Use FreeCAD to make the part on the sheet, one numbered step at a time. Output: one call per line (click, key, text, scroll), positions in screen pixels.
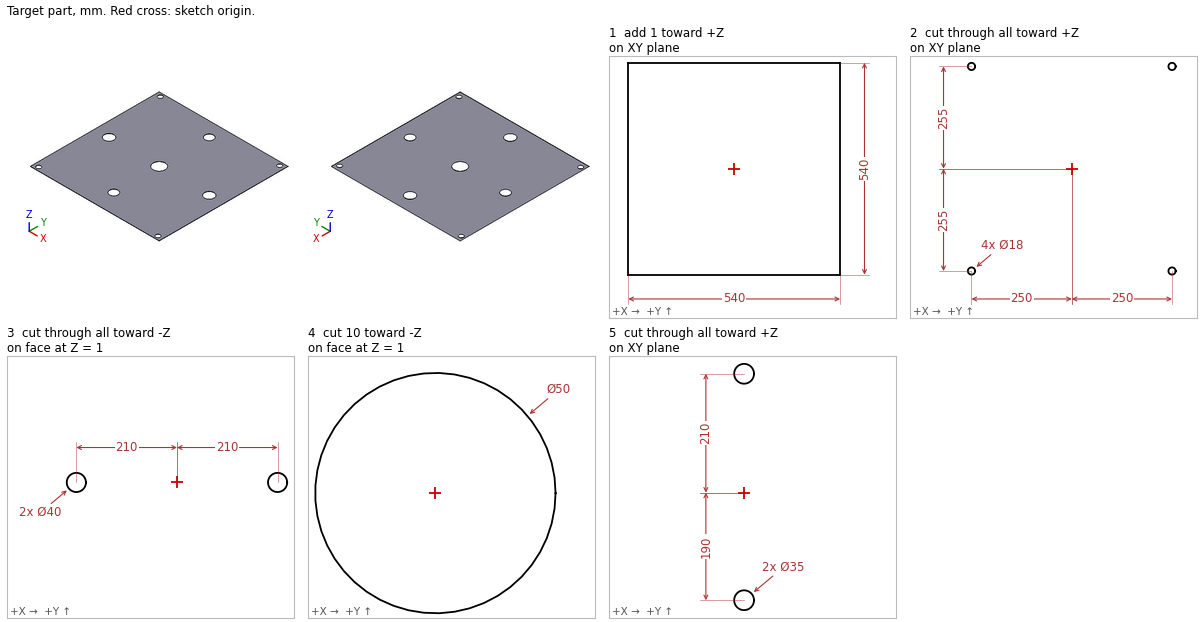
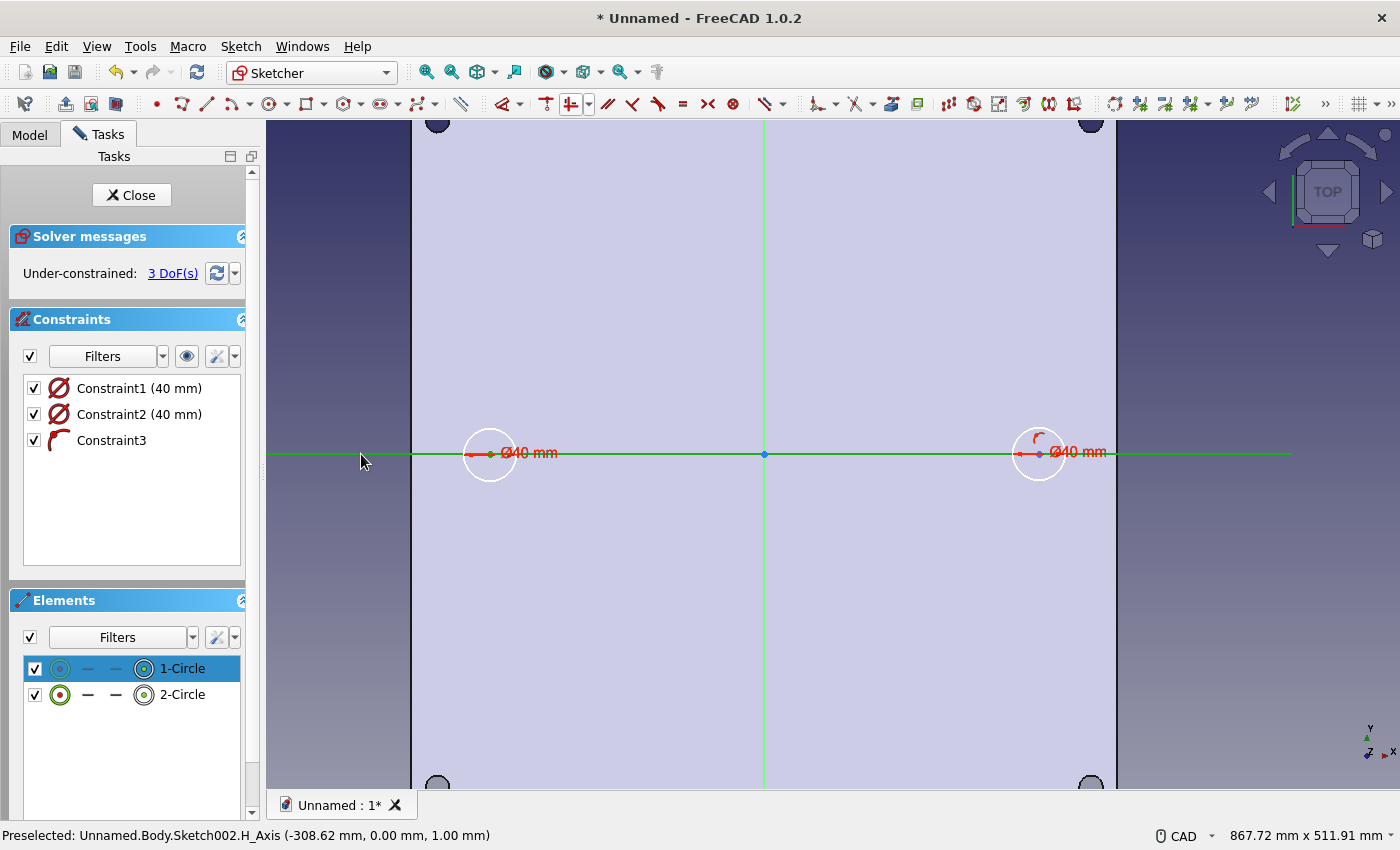
key(c)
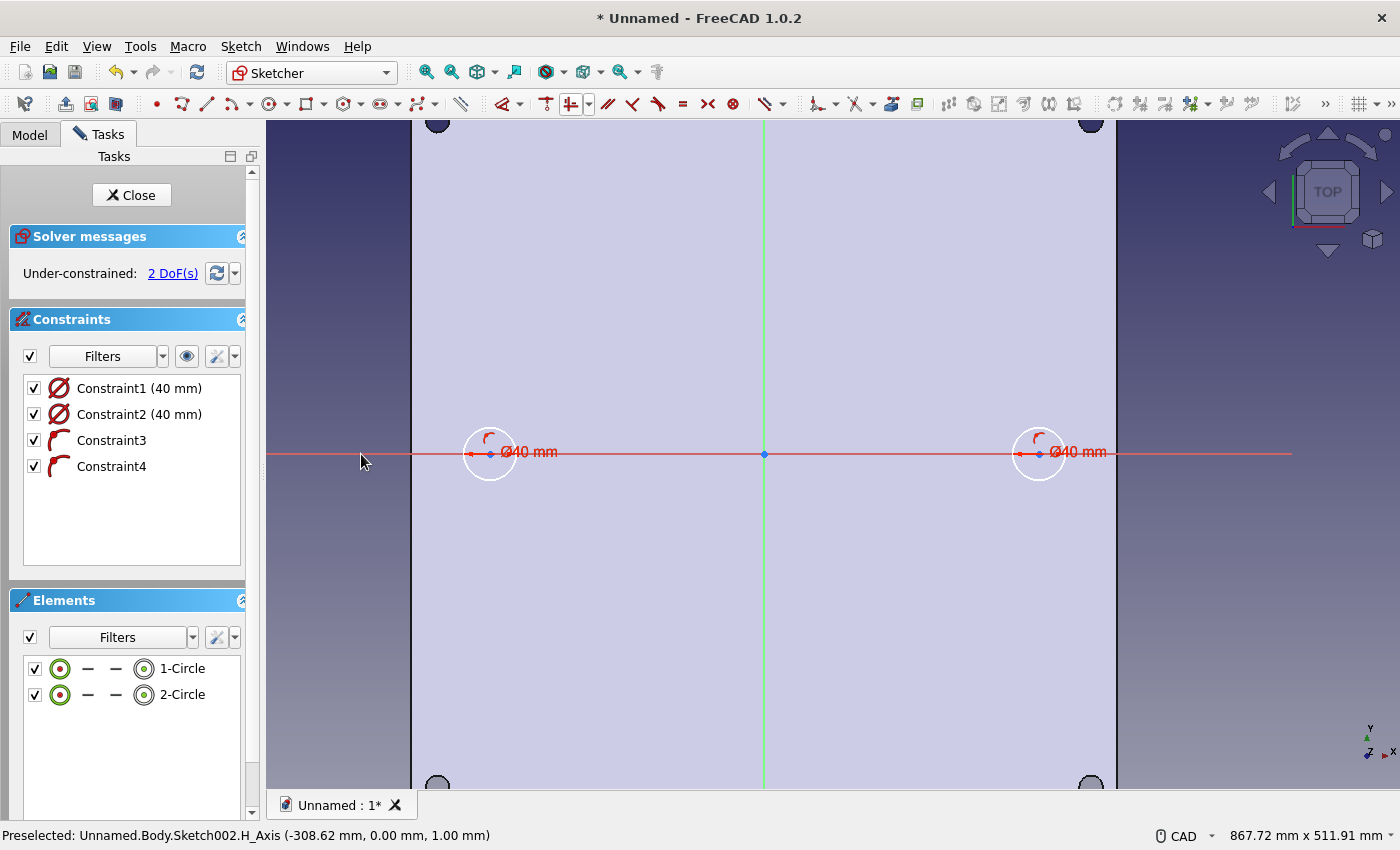
key(d)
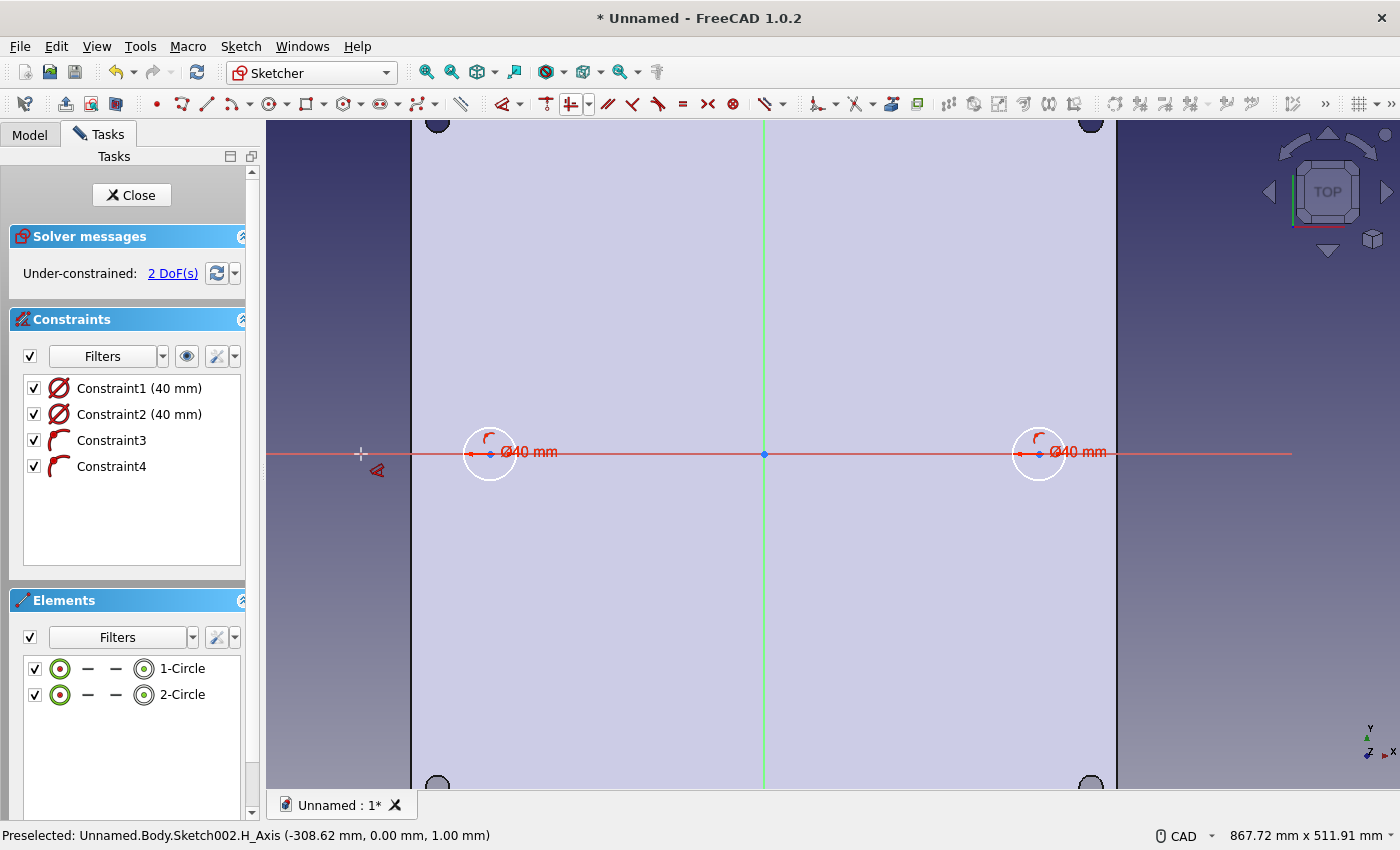
click(490, 454)
click(627, 488)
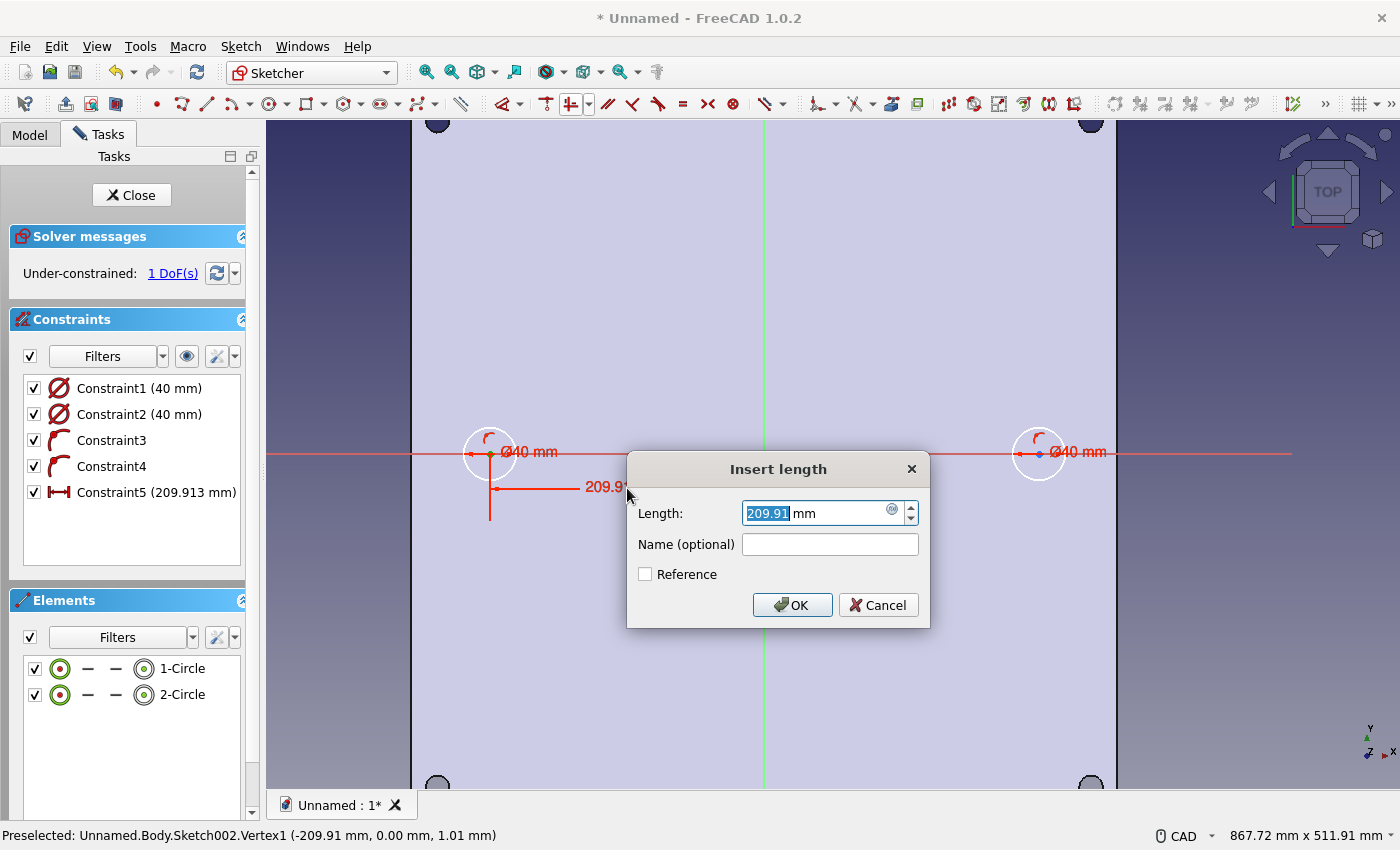
text(210)
key(Return)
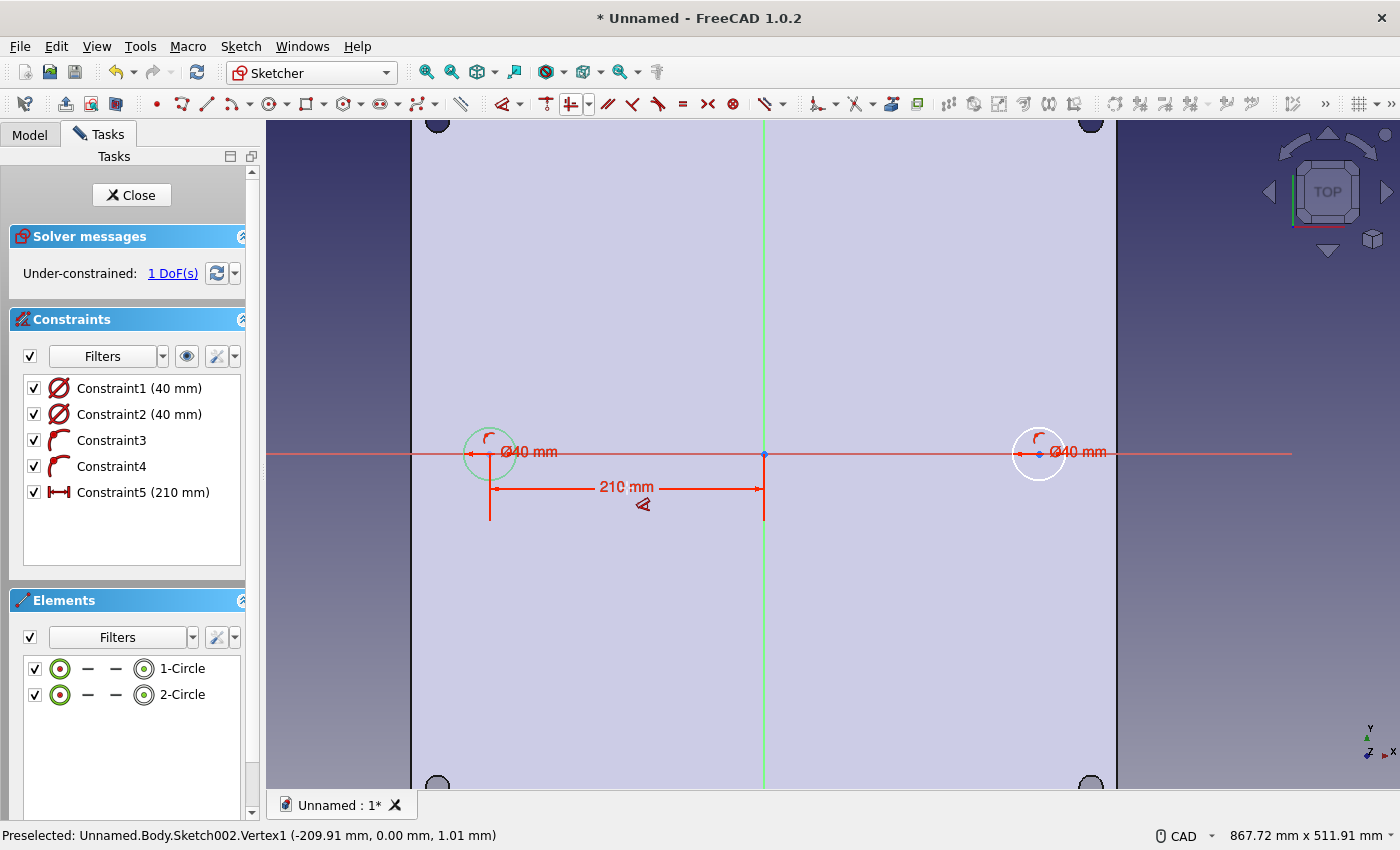
click(1039, 454)
click(902, 488)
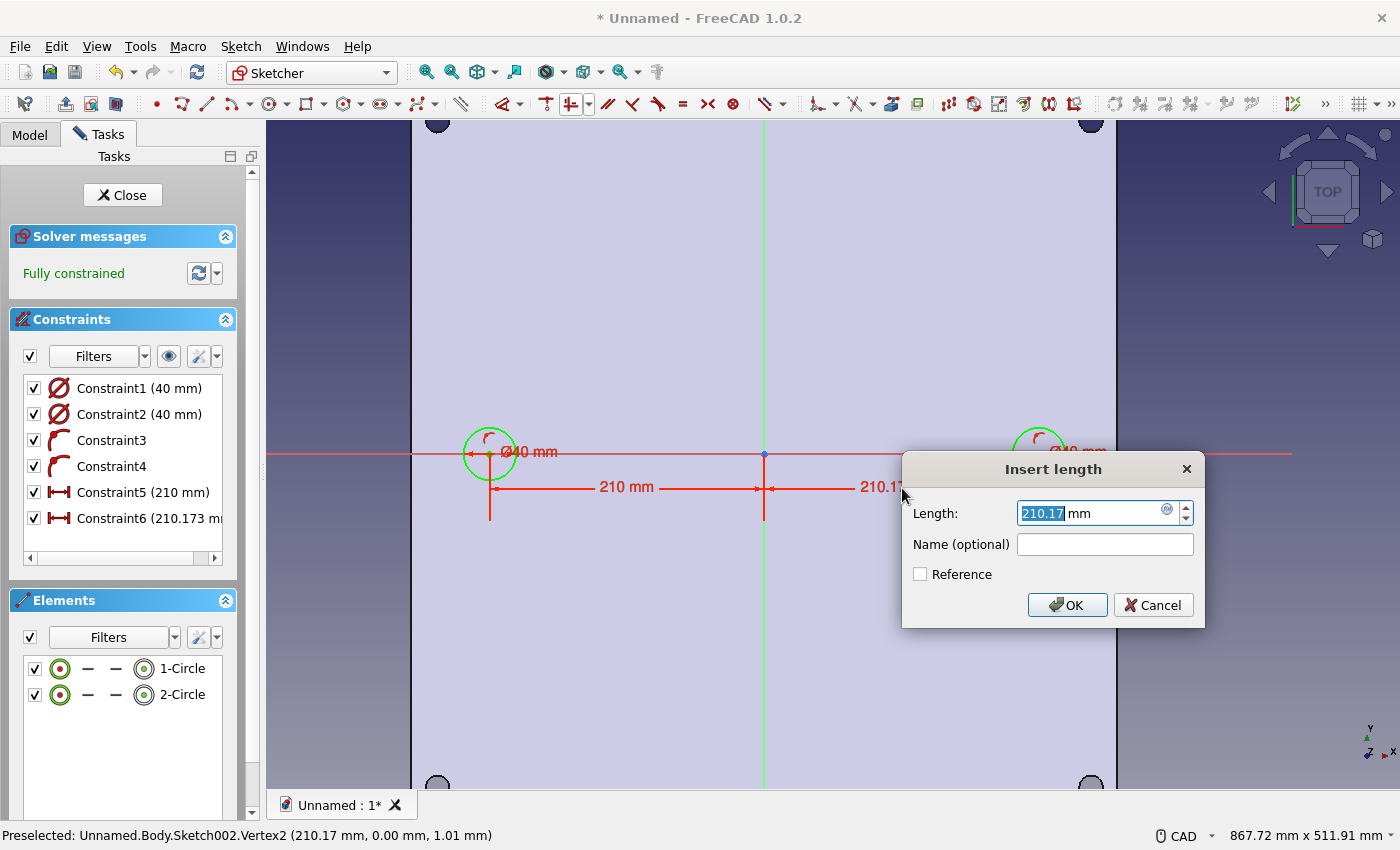
text(210)
key(Return)
key(Escape)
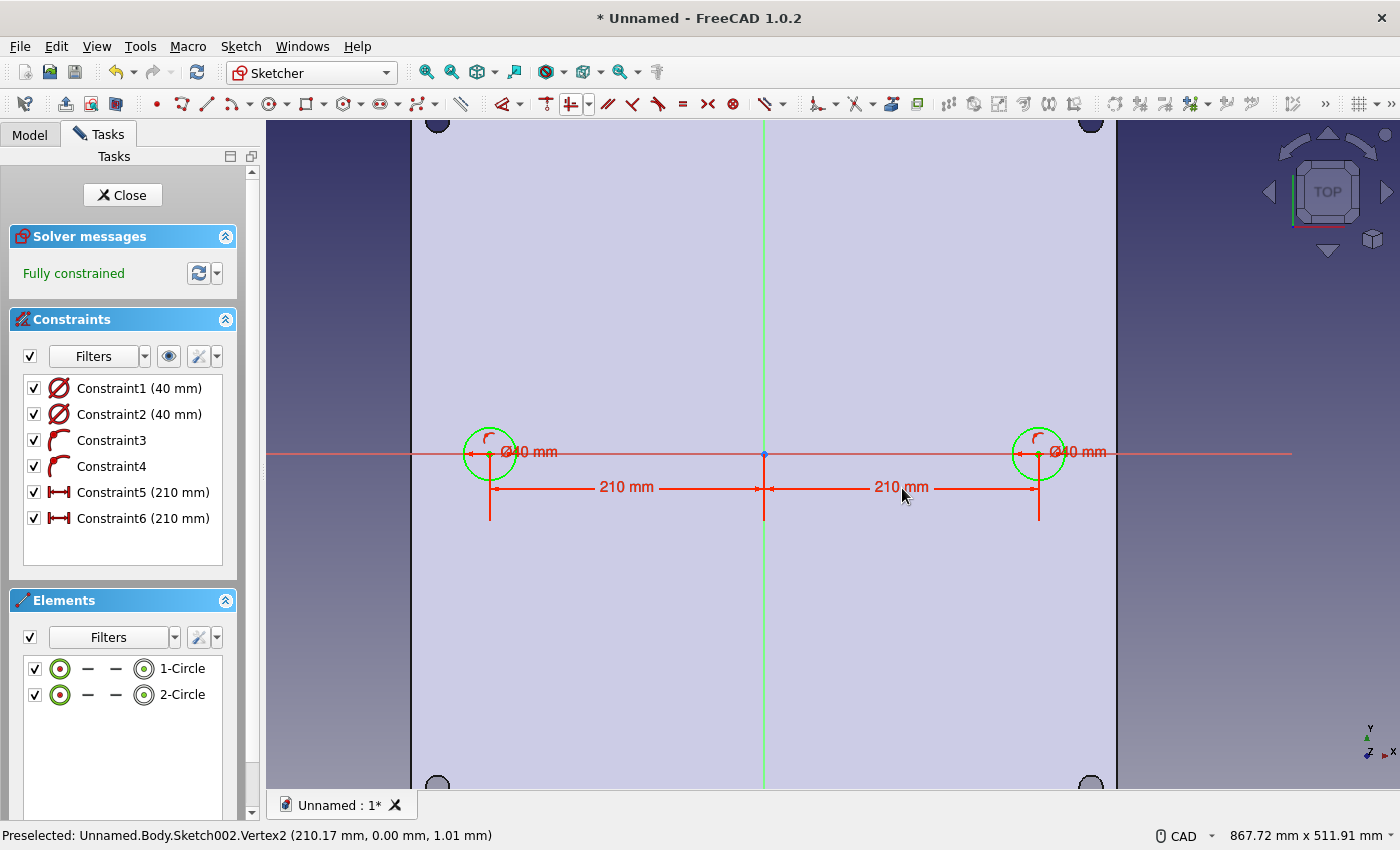
click(123, 195)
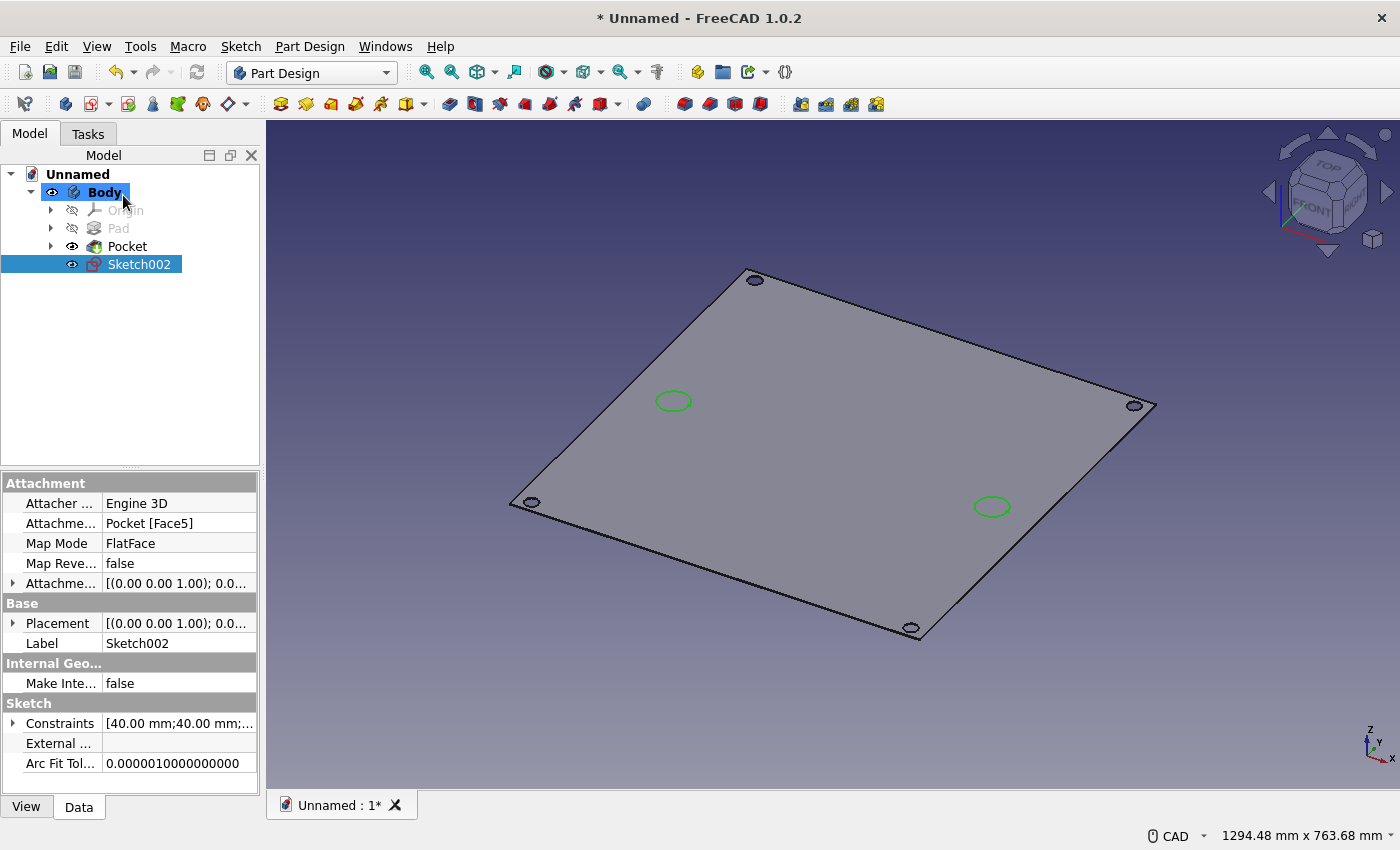
click(450, 104)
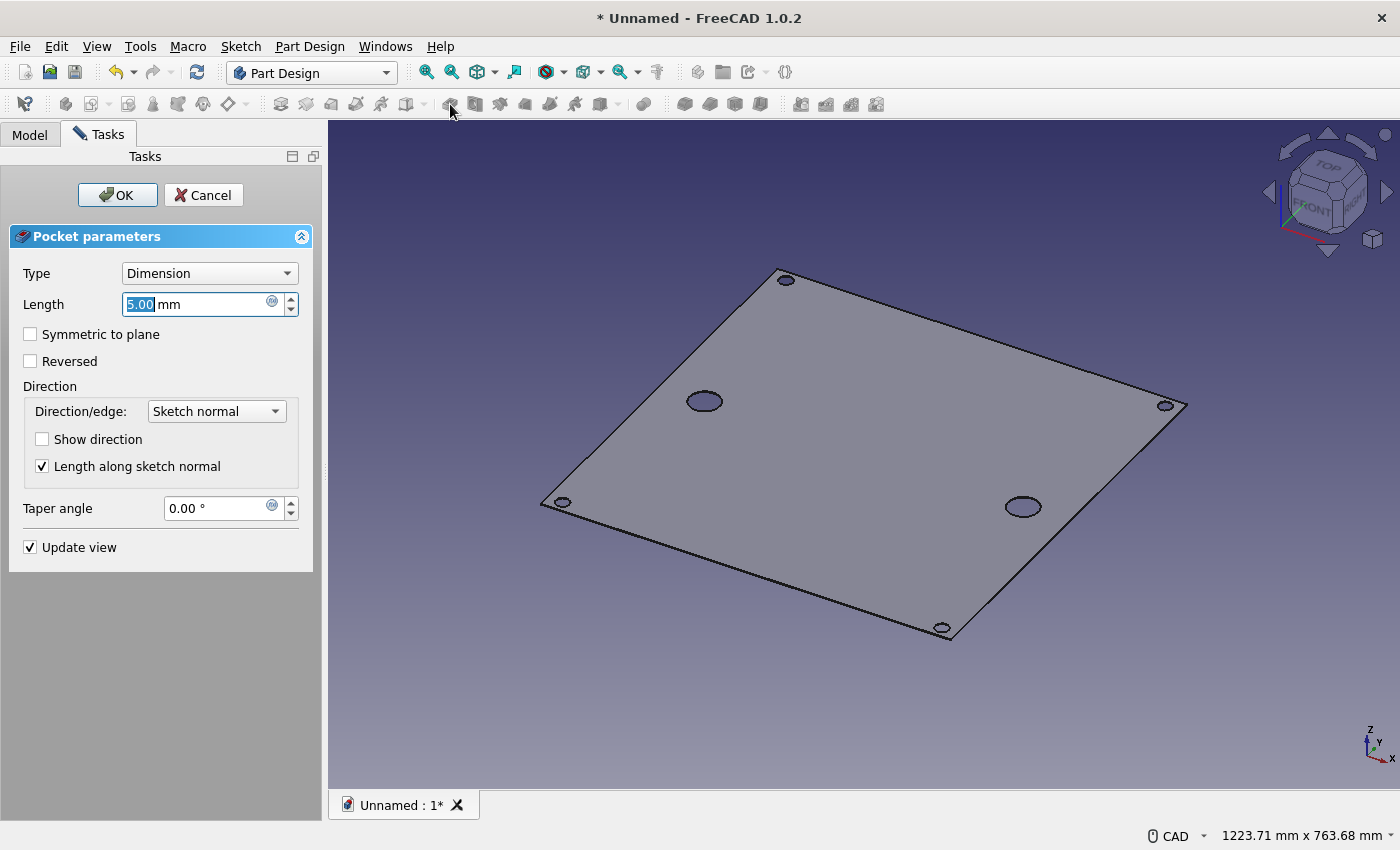
click(210, 274)